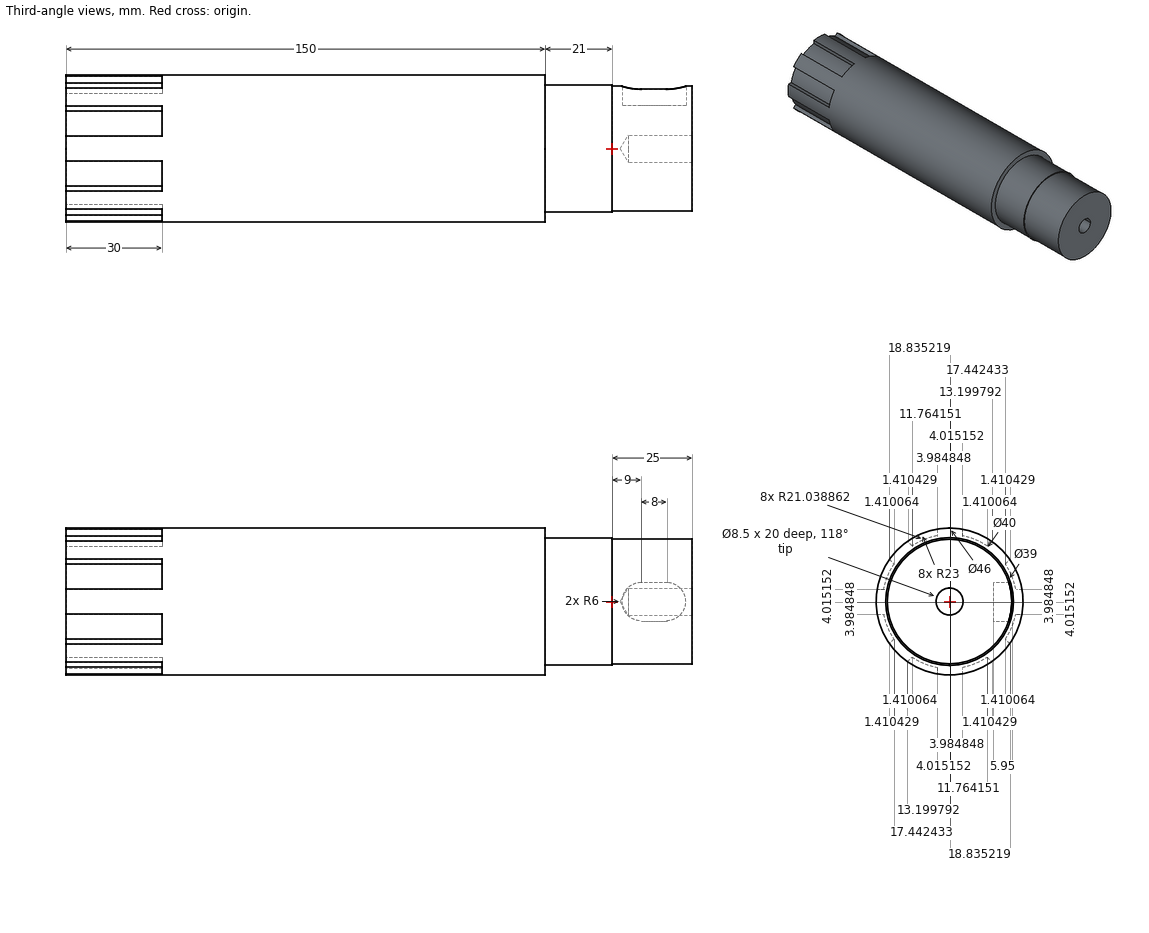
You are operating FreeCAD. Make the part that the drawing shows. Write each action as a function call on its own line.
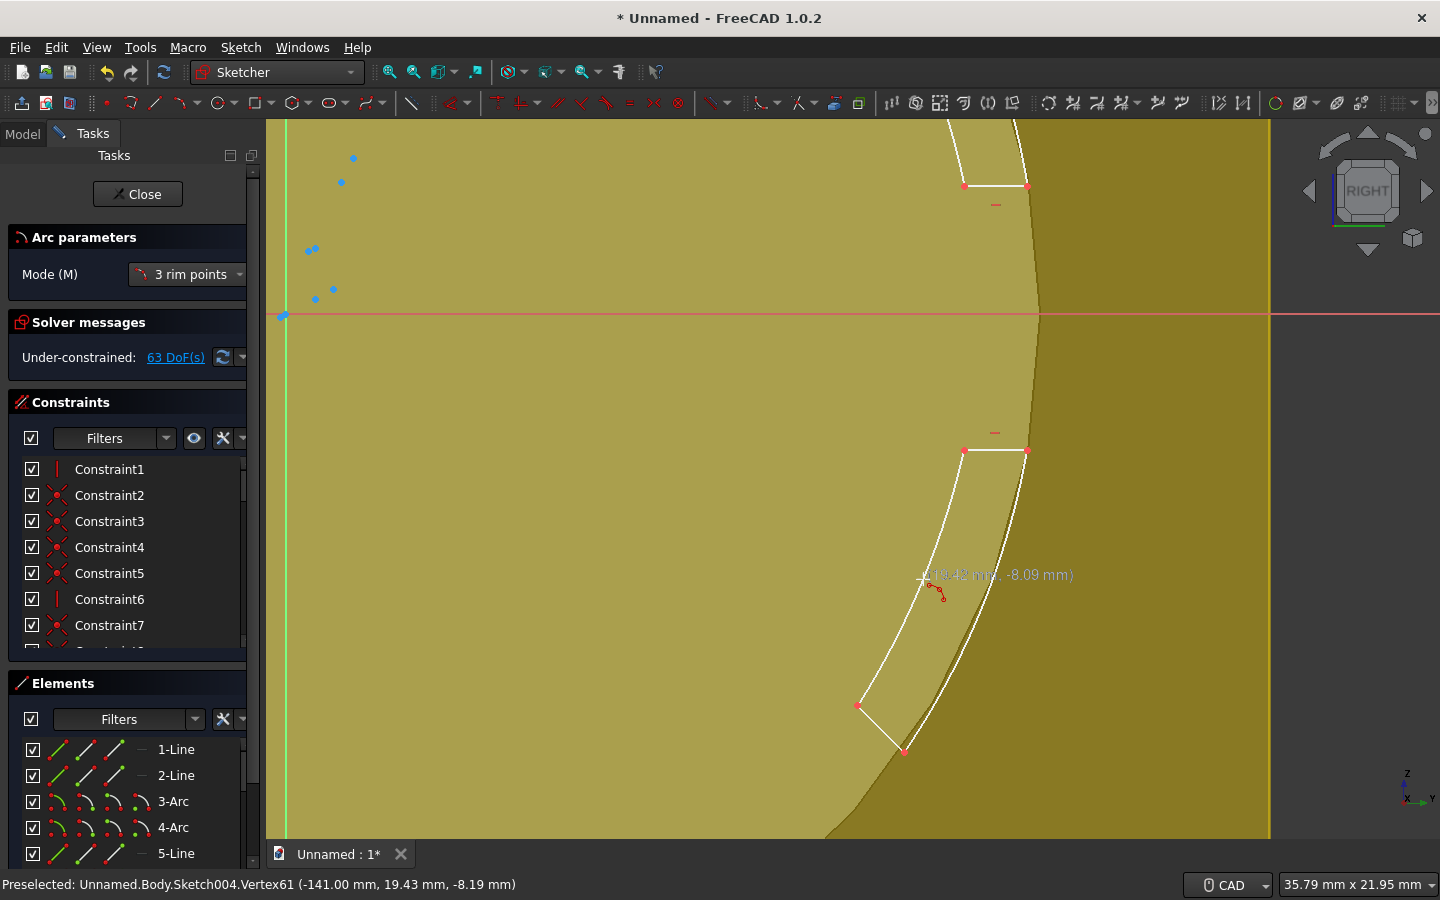
click(156, 104)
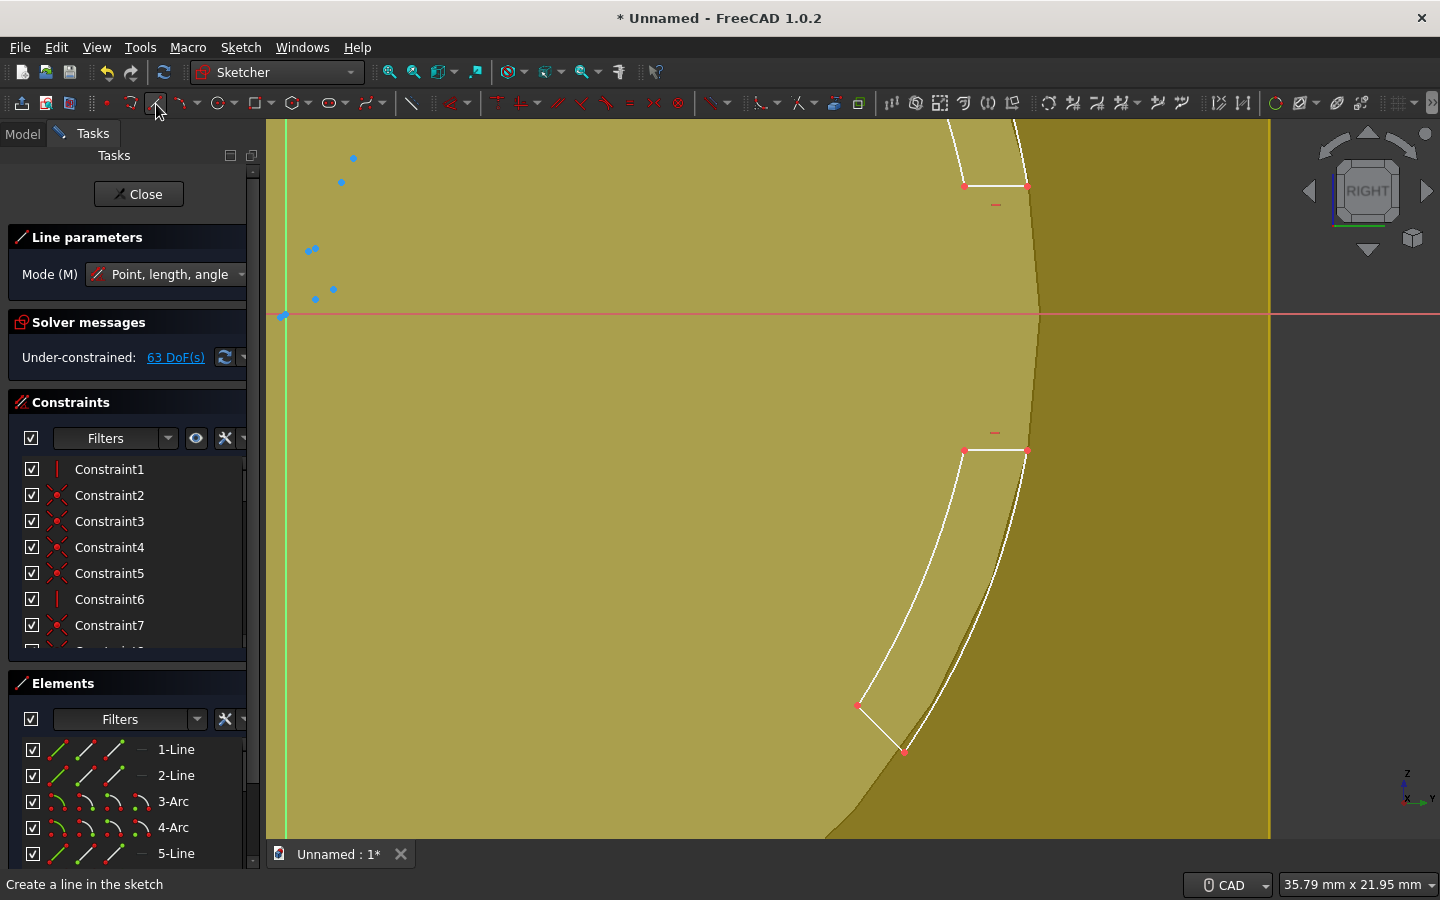
scroll(999, 550, down, 6)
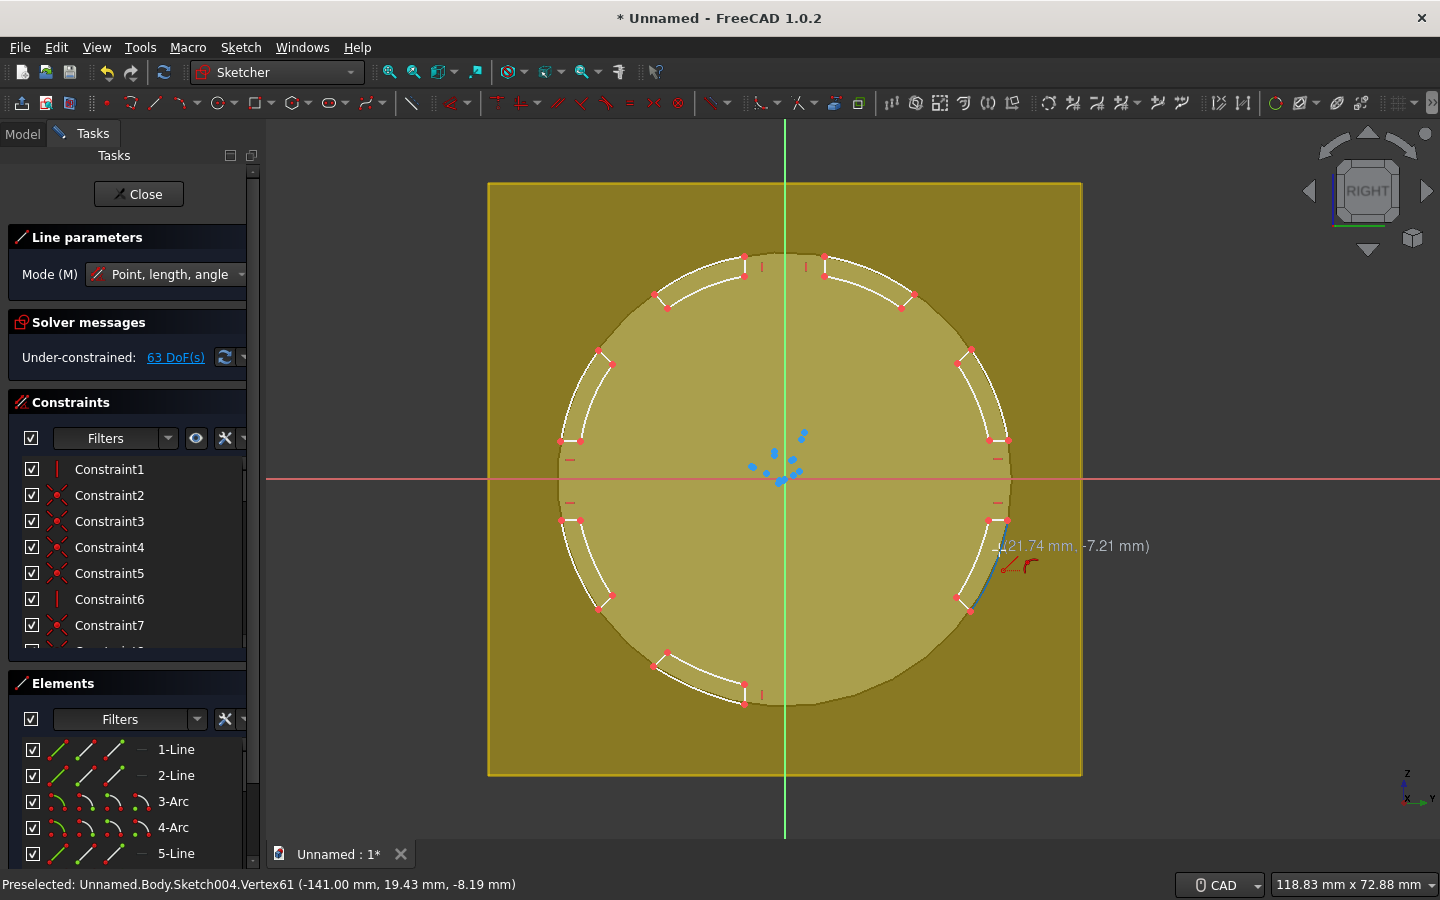
click(901, 652)
click(915, 666)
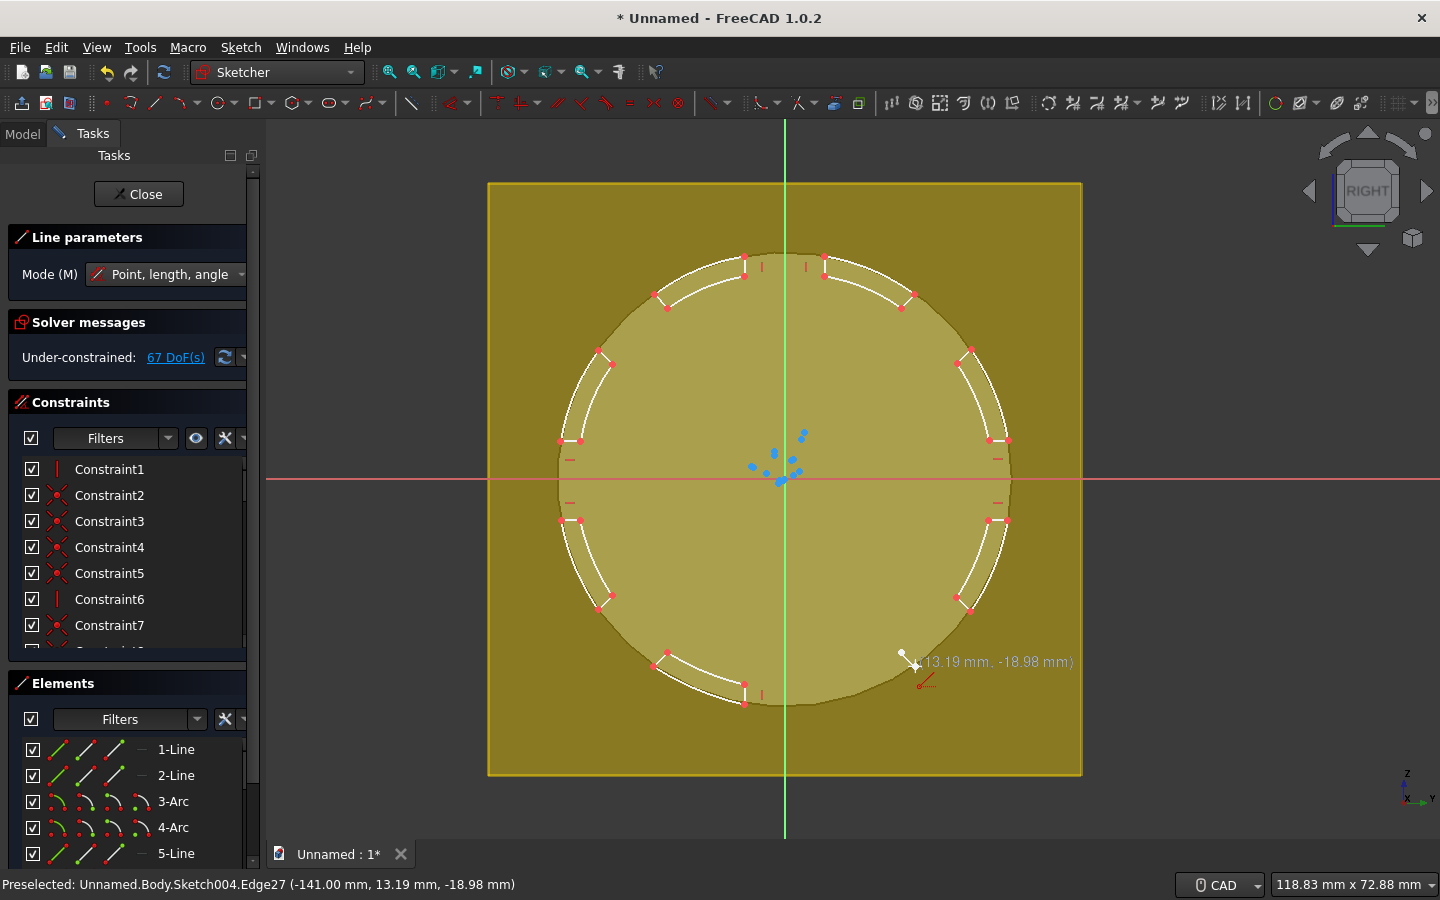
click(824, 703)
click(824, 684)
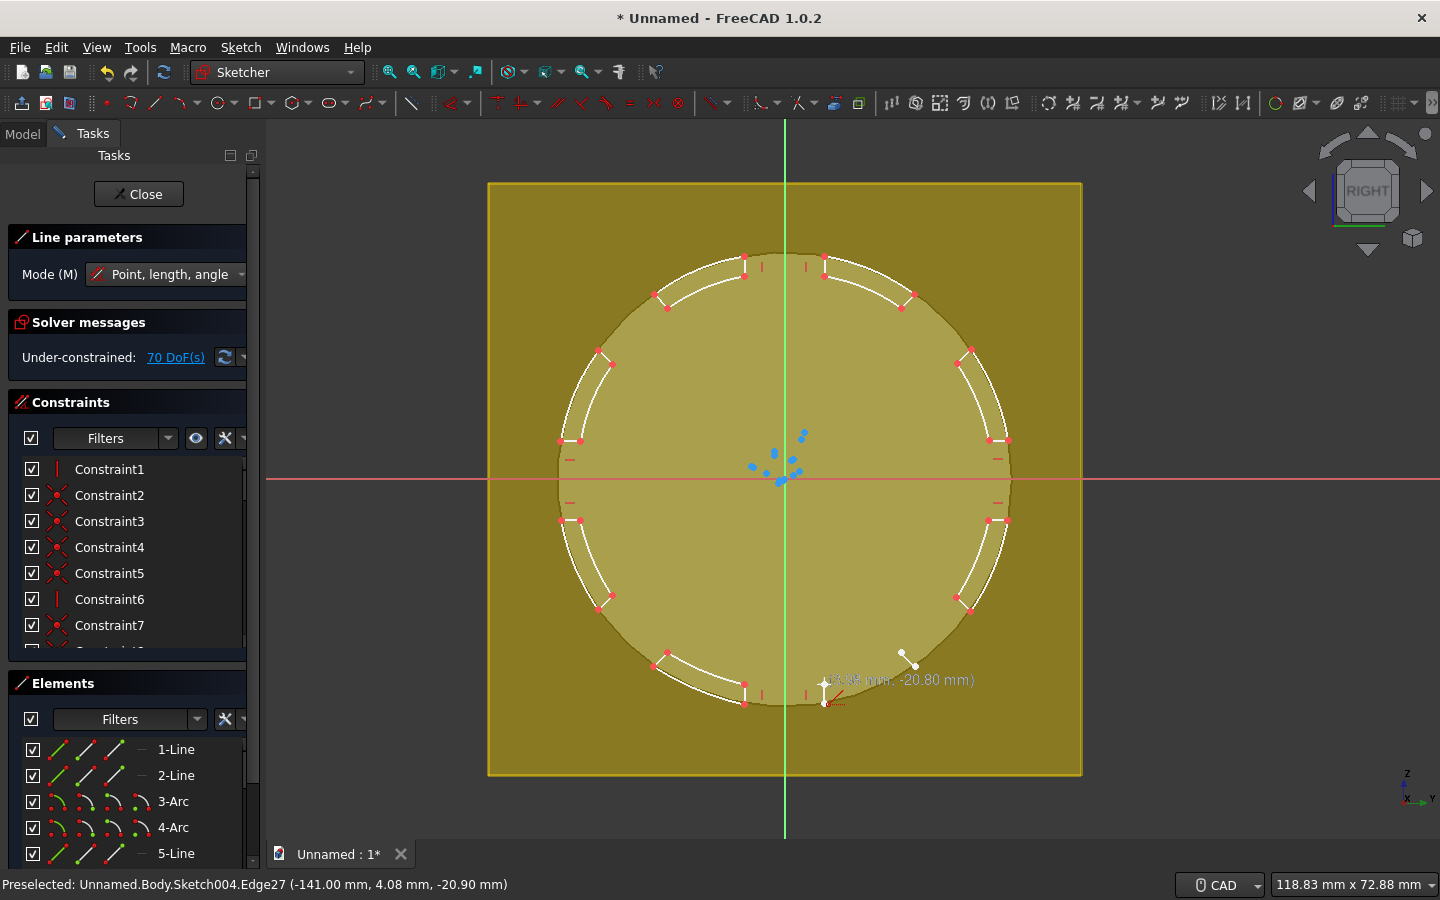
click(180, 104)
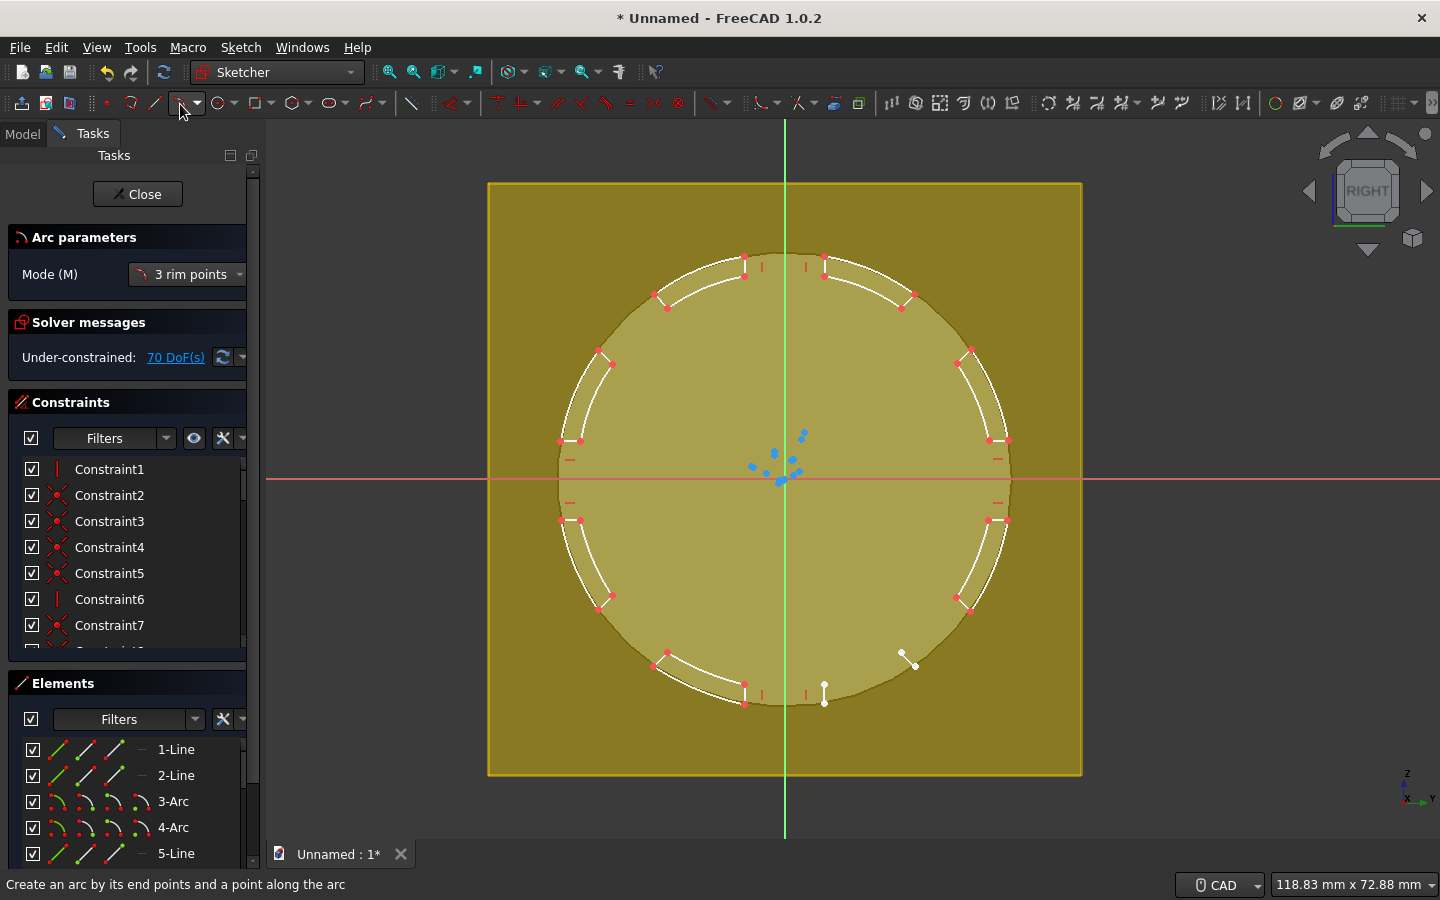
scroll(915, 666, up, 3)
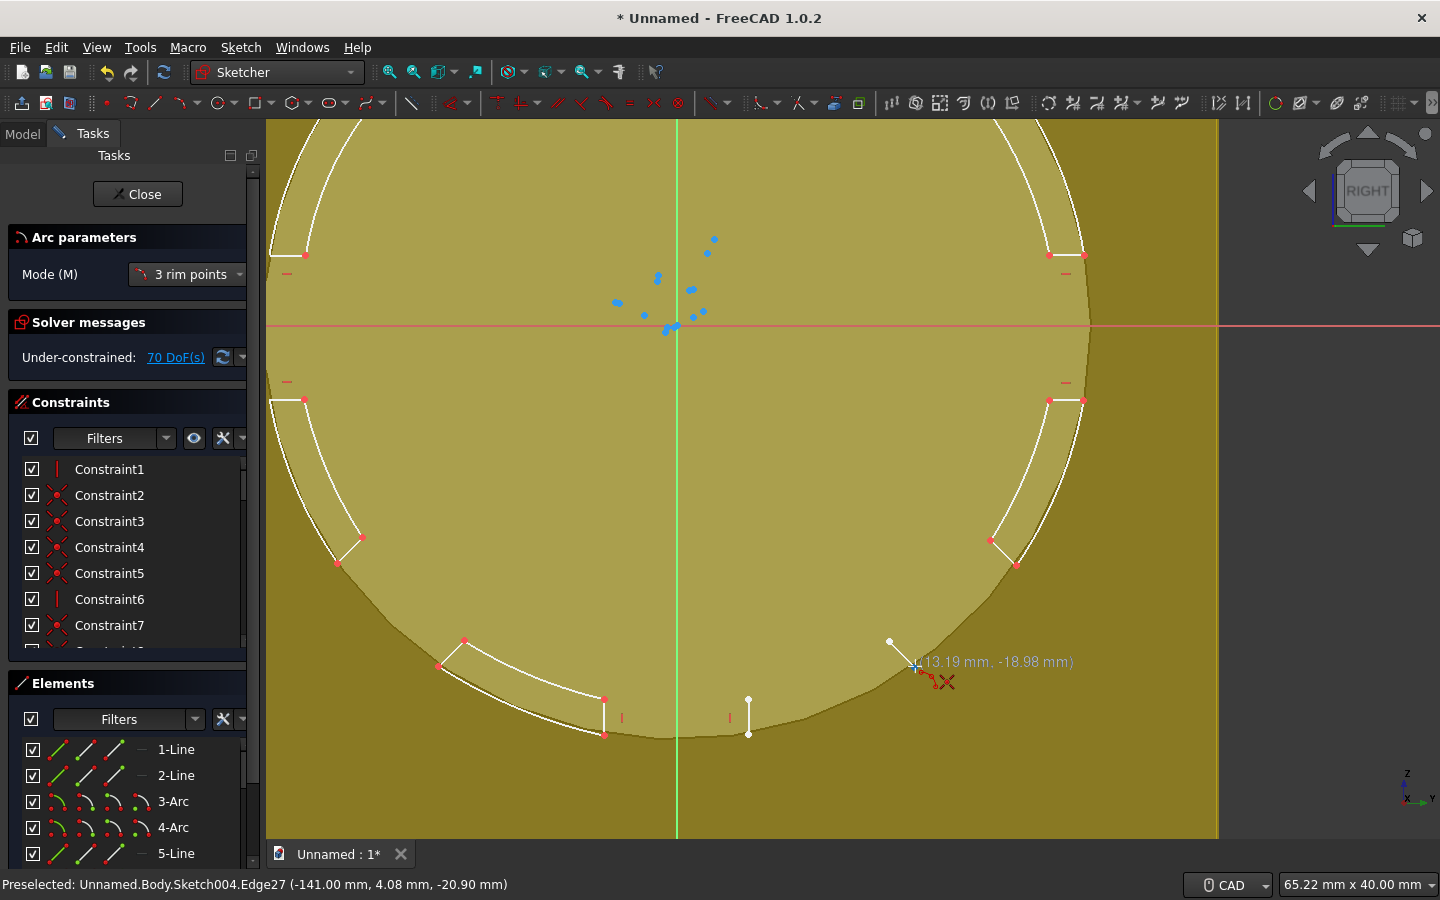
click(915, 667)
click(749, 735)